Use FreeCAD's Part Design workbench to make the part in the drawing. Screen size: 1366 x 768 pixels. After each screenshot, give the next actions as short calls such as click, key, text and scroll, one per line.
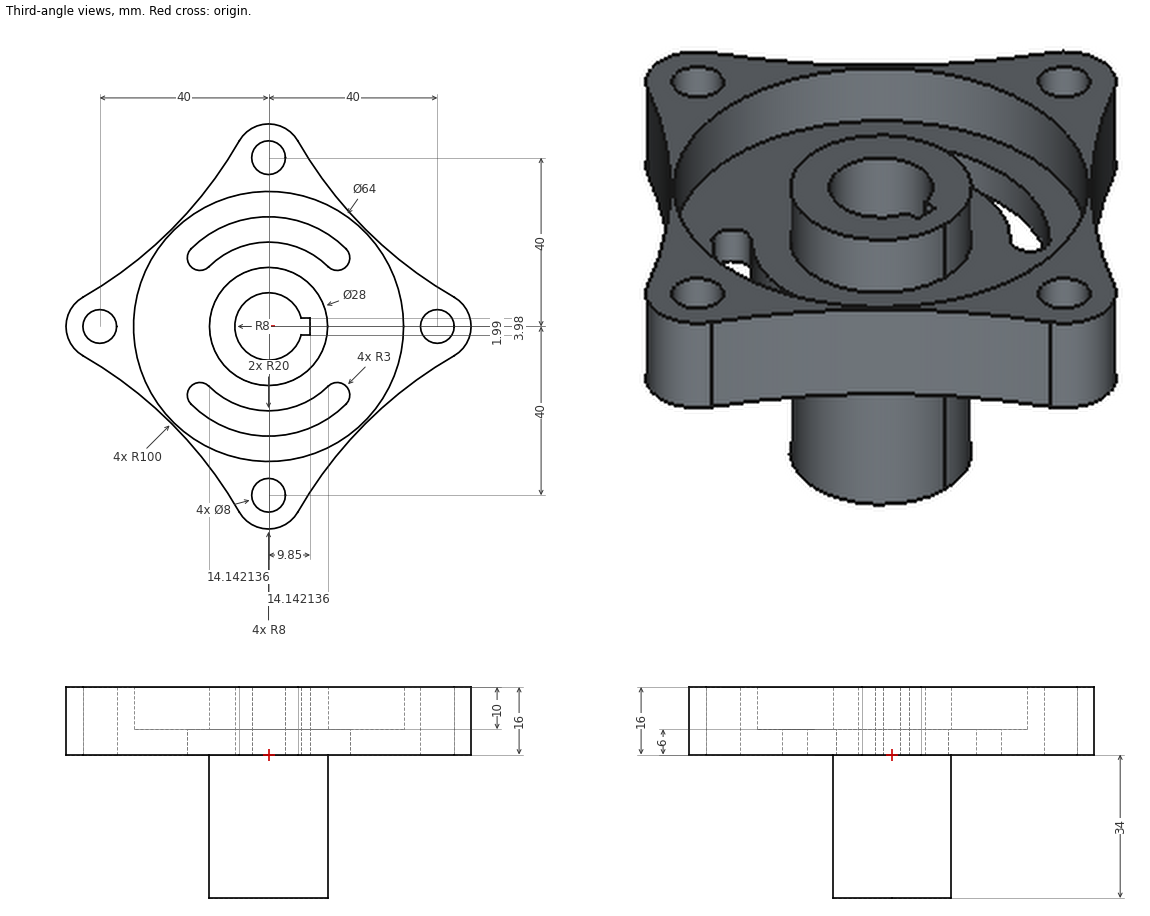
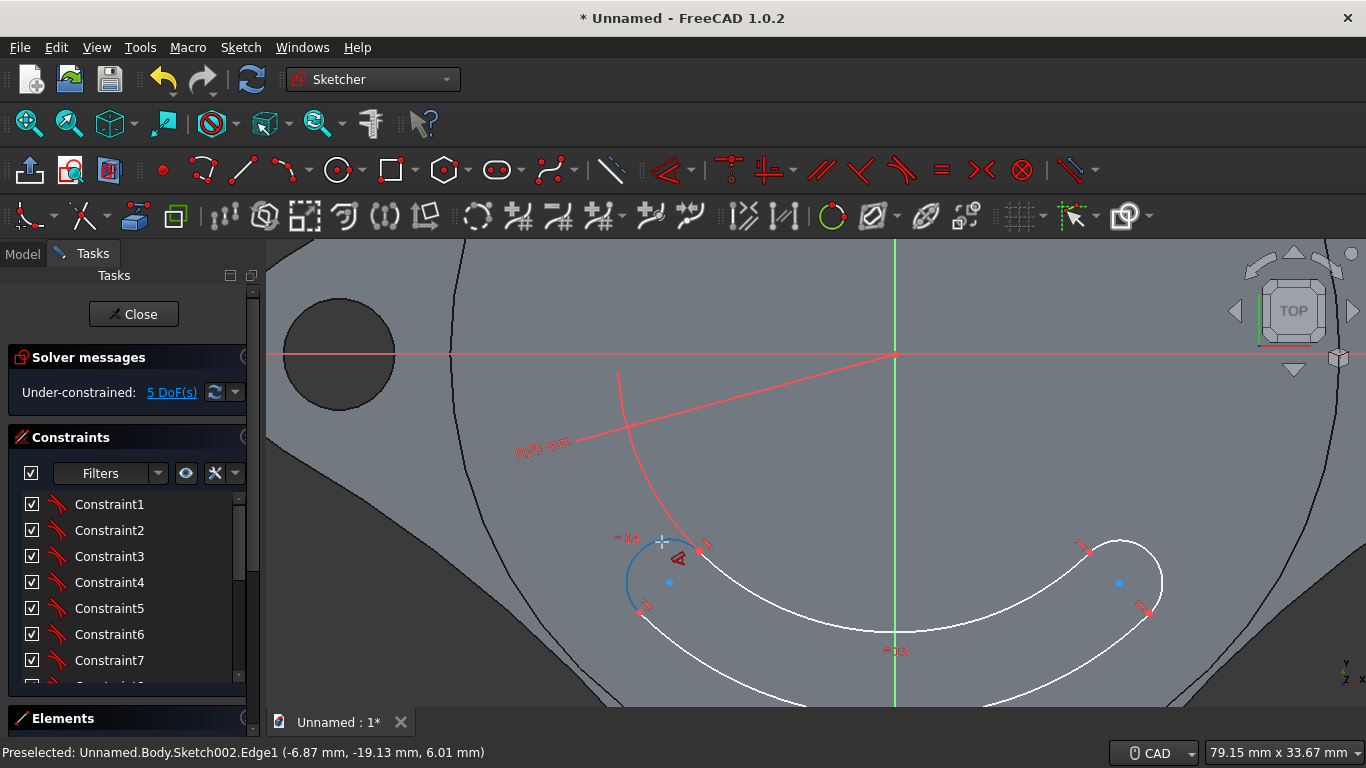
click(662, 540)
click(657, 508)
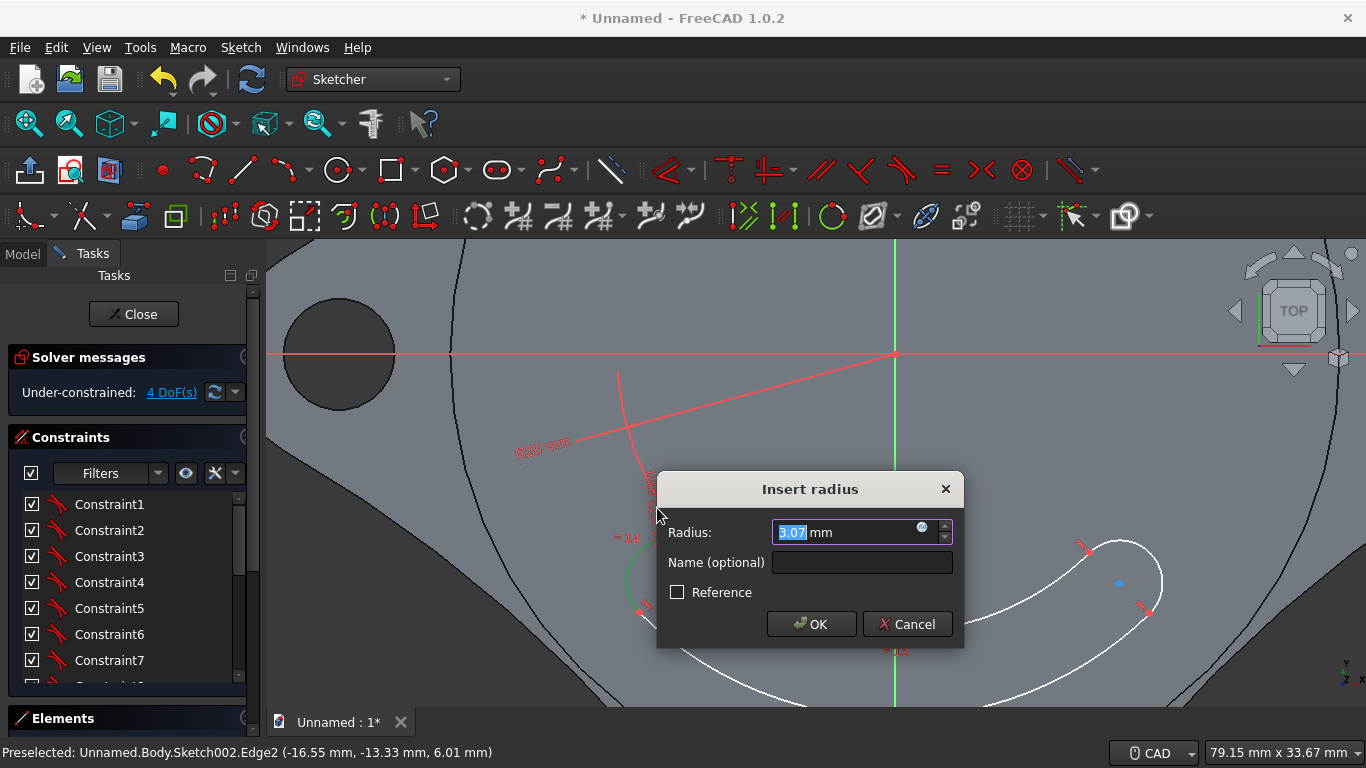
text(3)
key(Return)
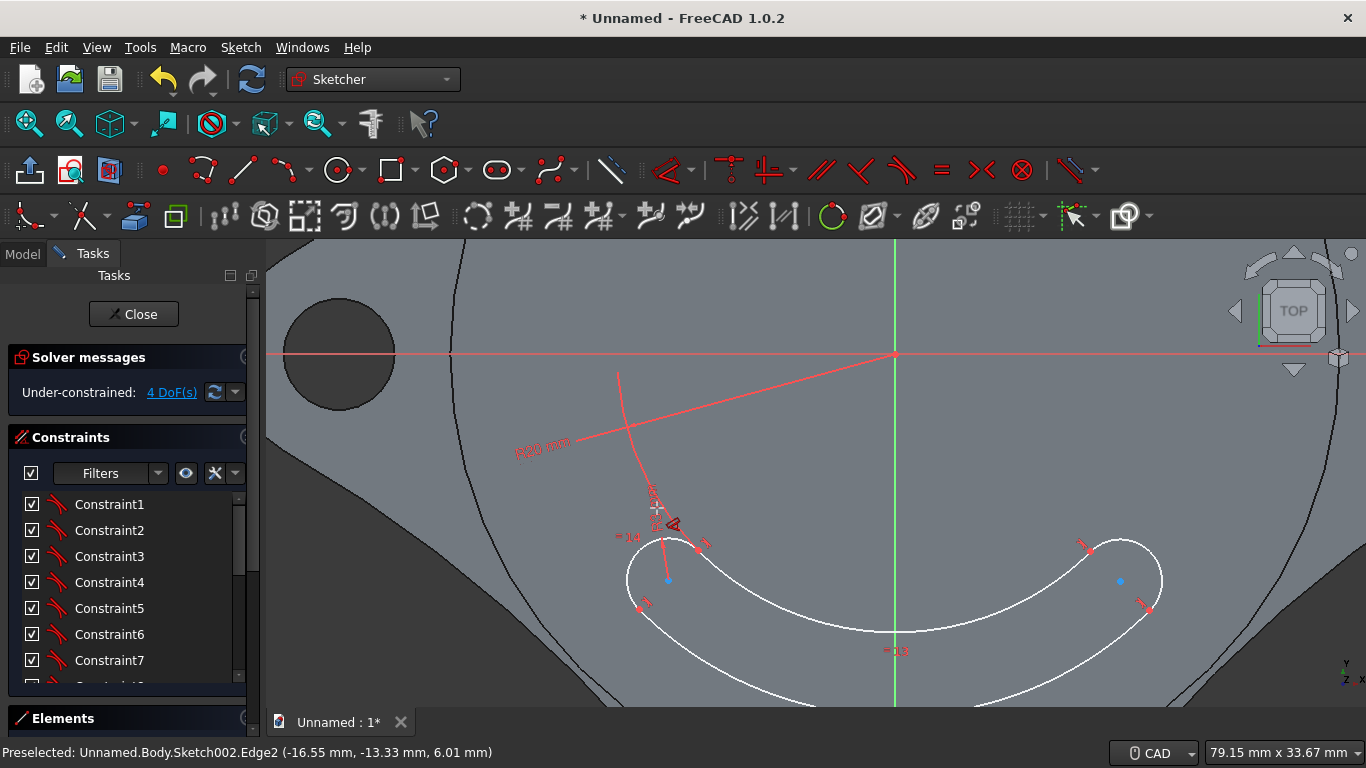
click(698, 551)
click(797, 585)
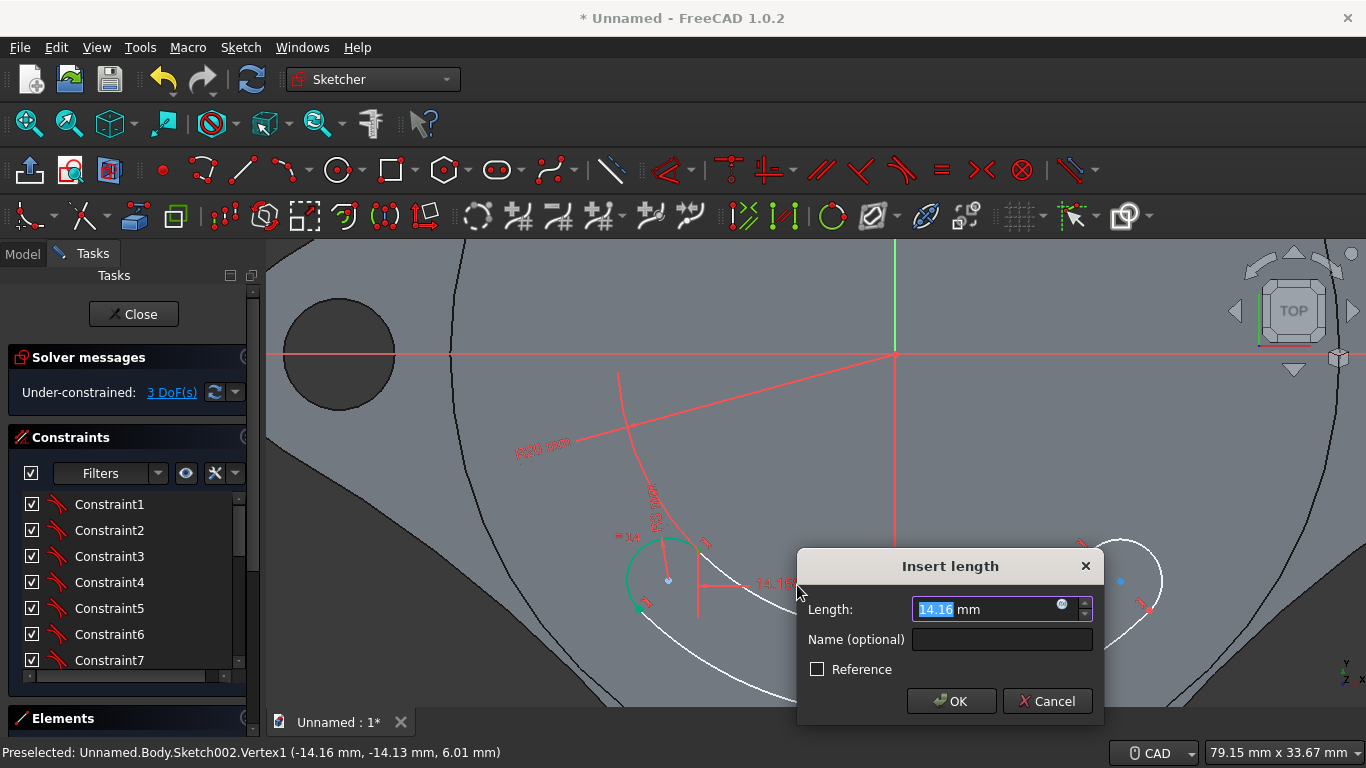
text(14.142136)
key(Return)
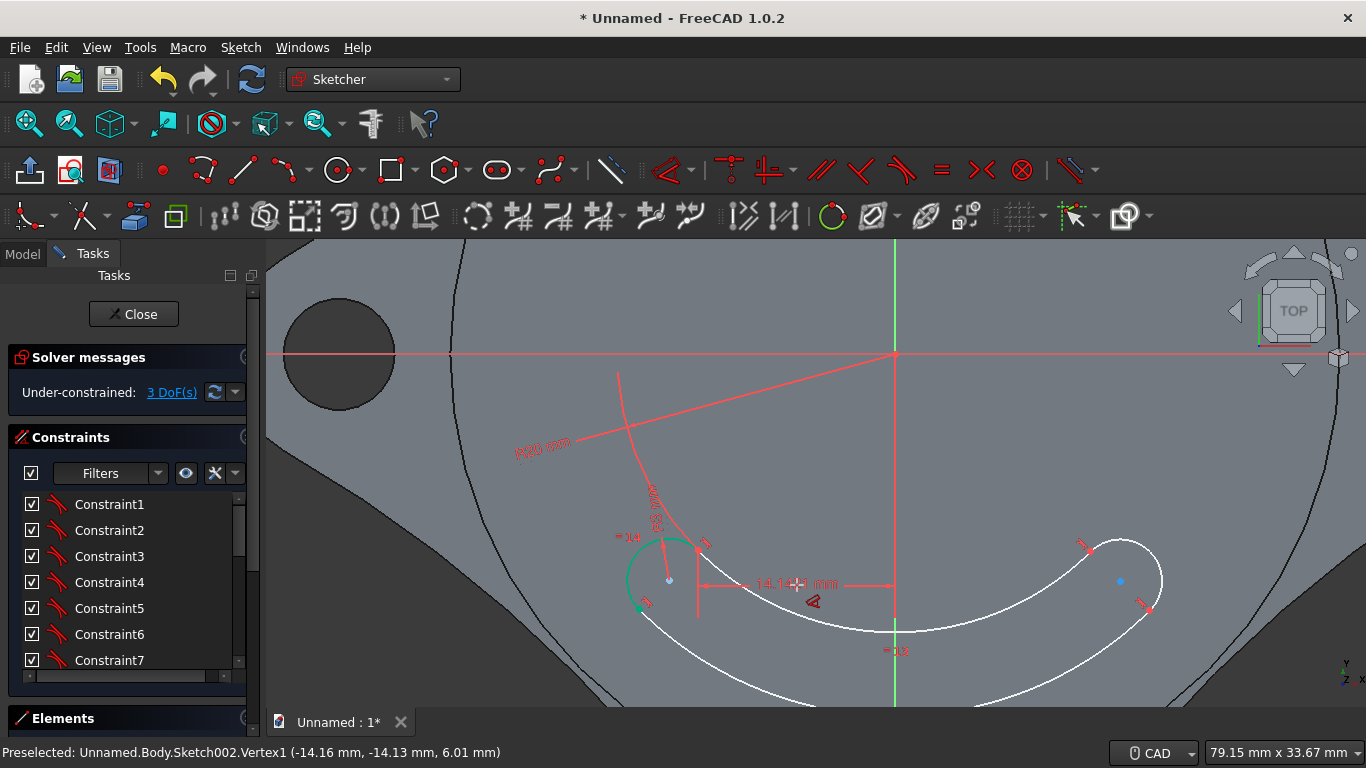
click(1091, 552)
click(993, 586)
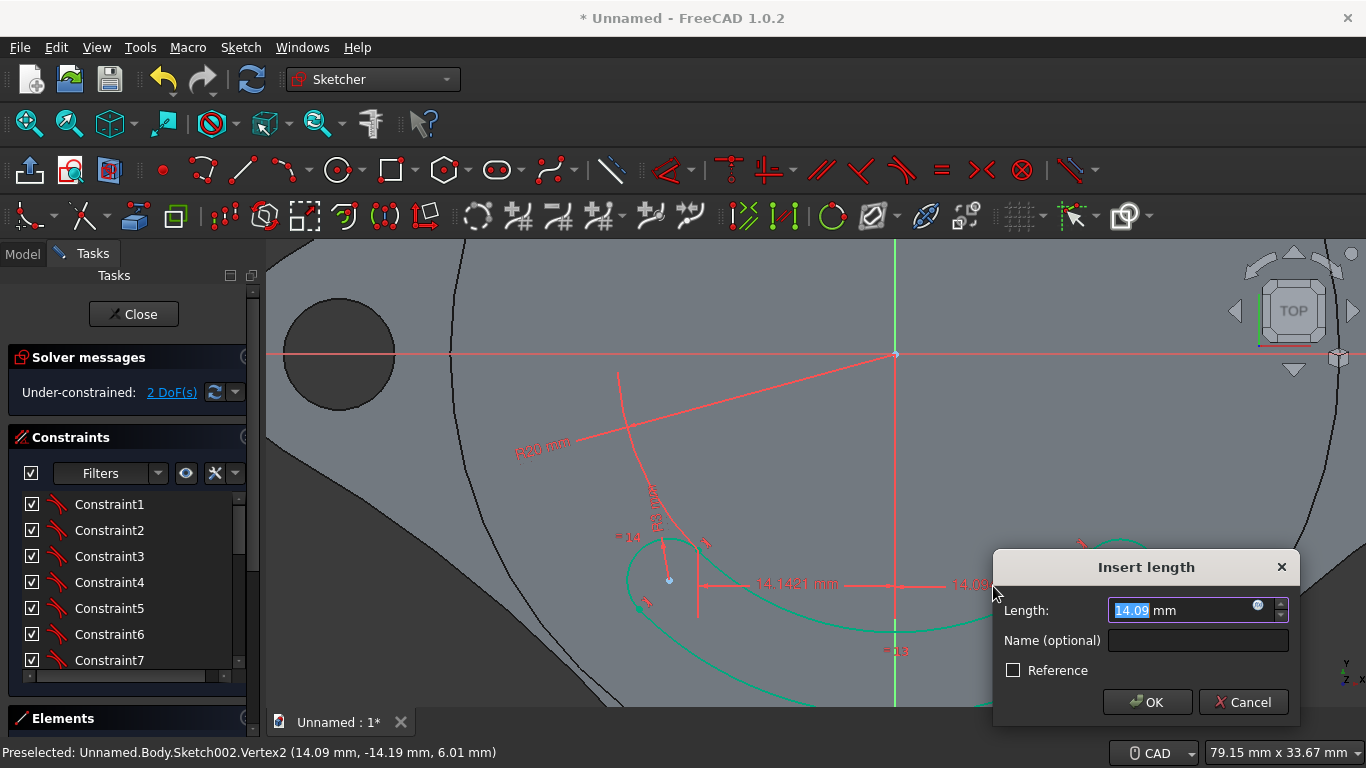
text(14.142136)
key(Return)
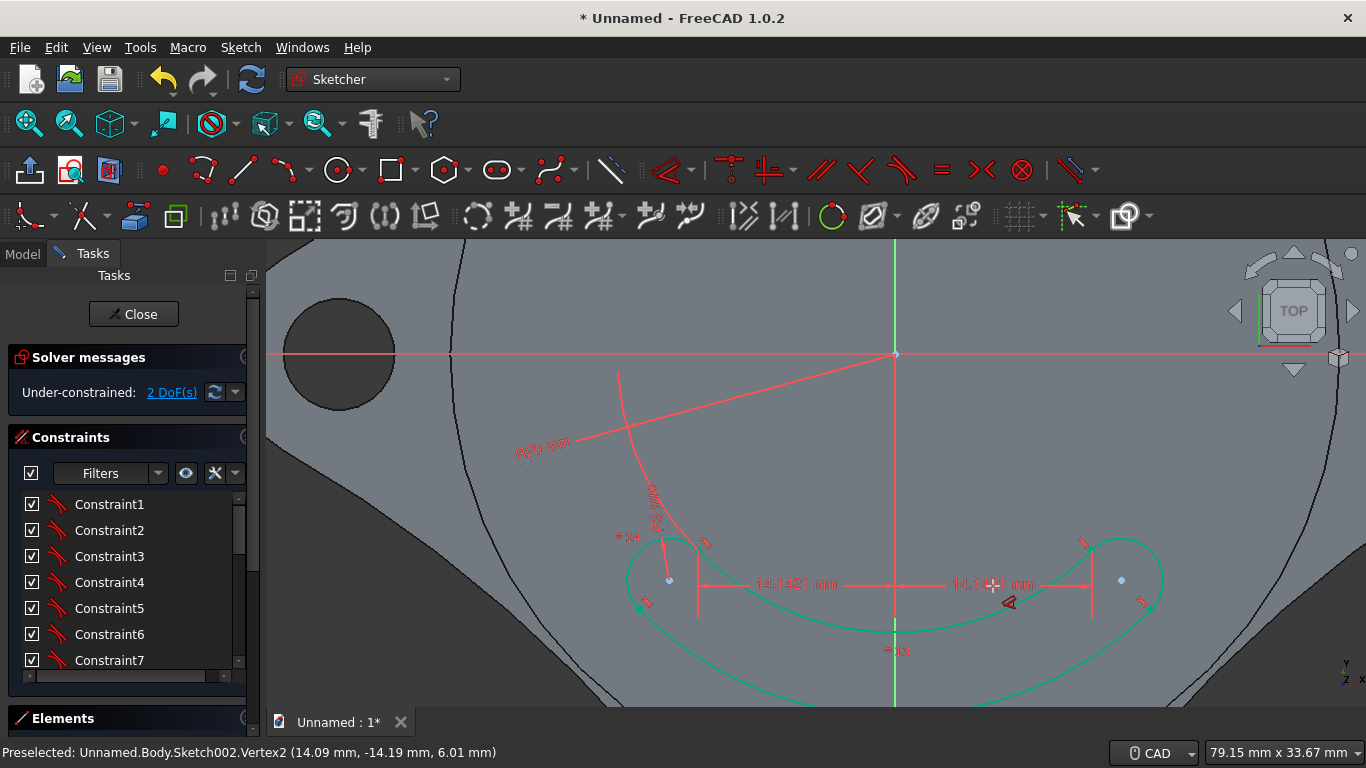
scroll(662, 542, down, 5)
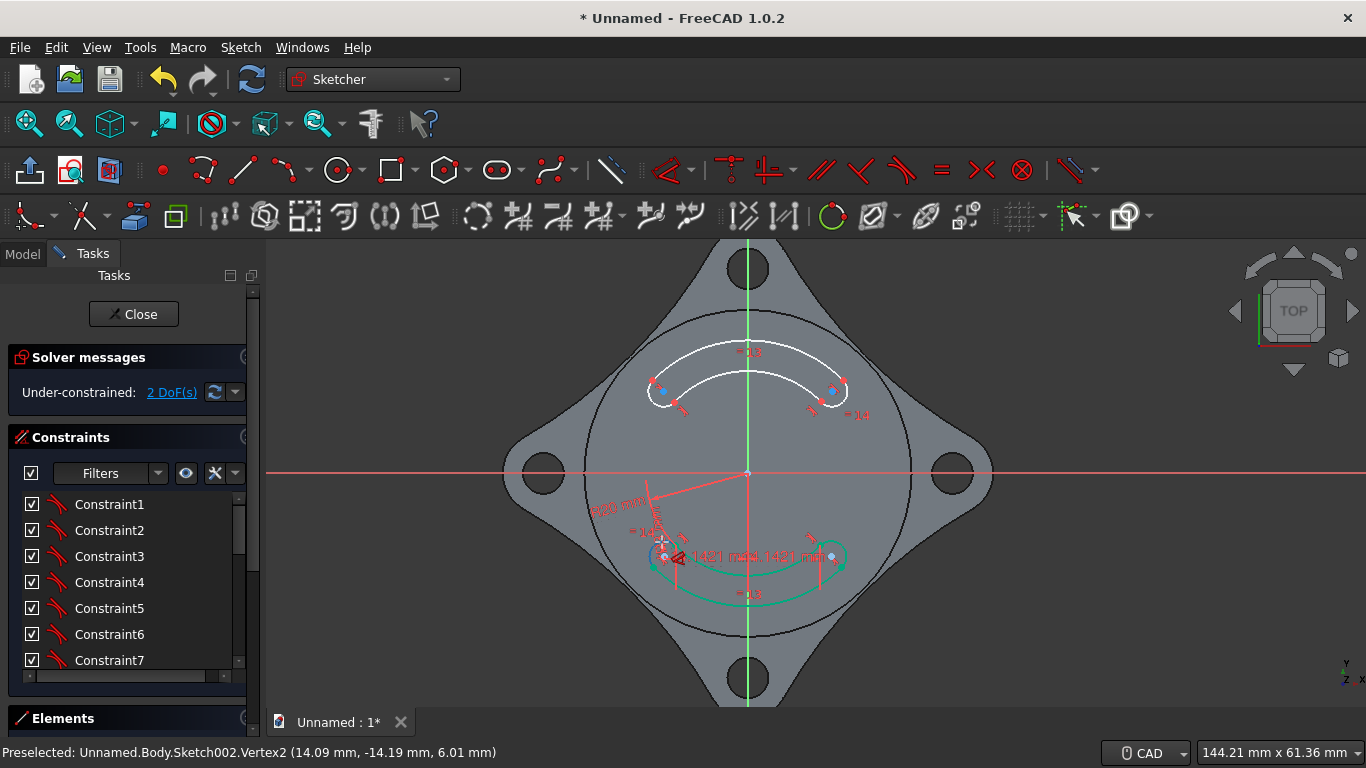
click(821, 402)
click(801, 368)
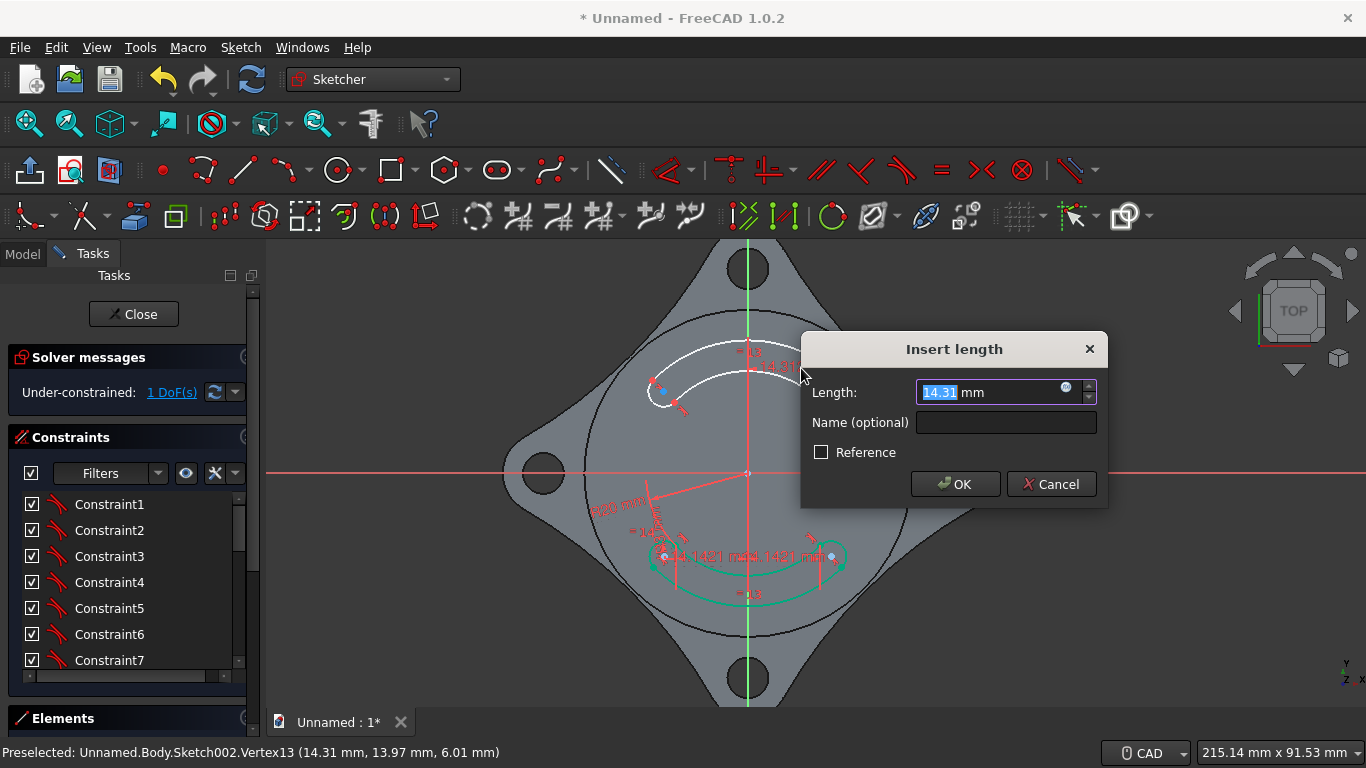
text(14.142136)
key(Return)